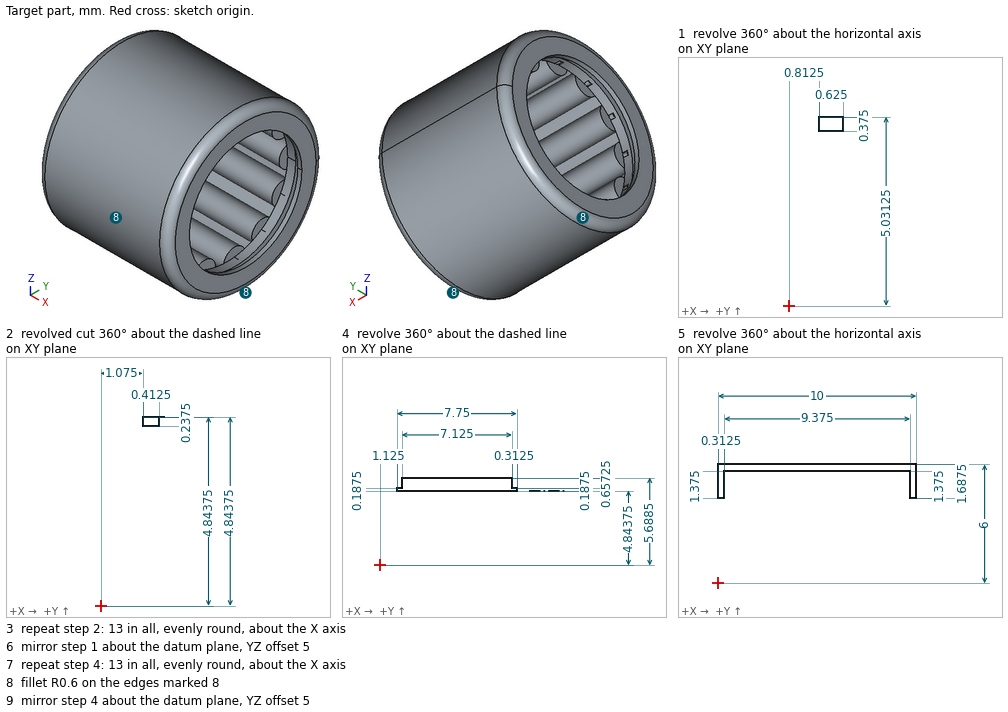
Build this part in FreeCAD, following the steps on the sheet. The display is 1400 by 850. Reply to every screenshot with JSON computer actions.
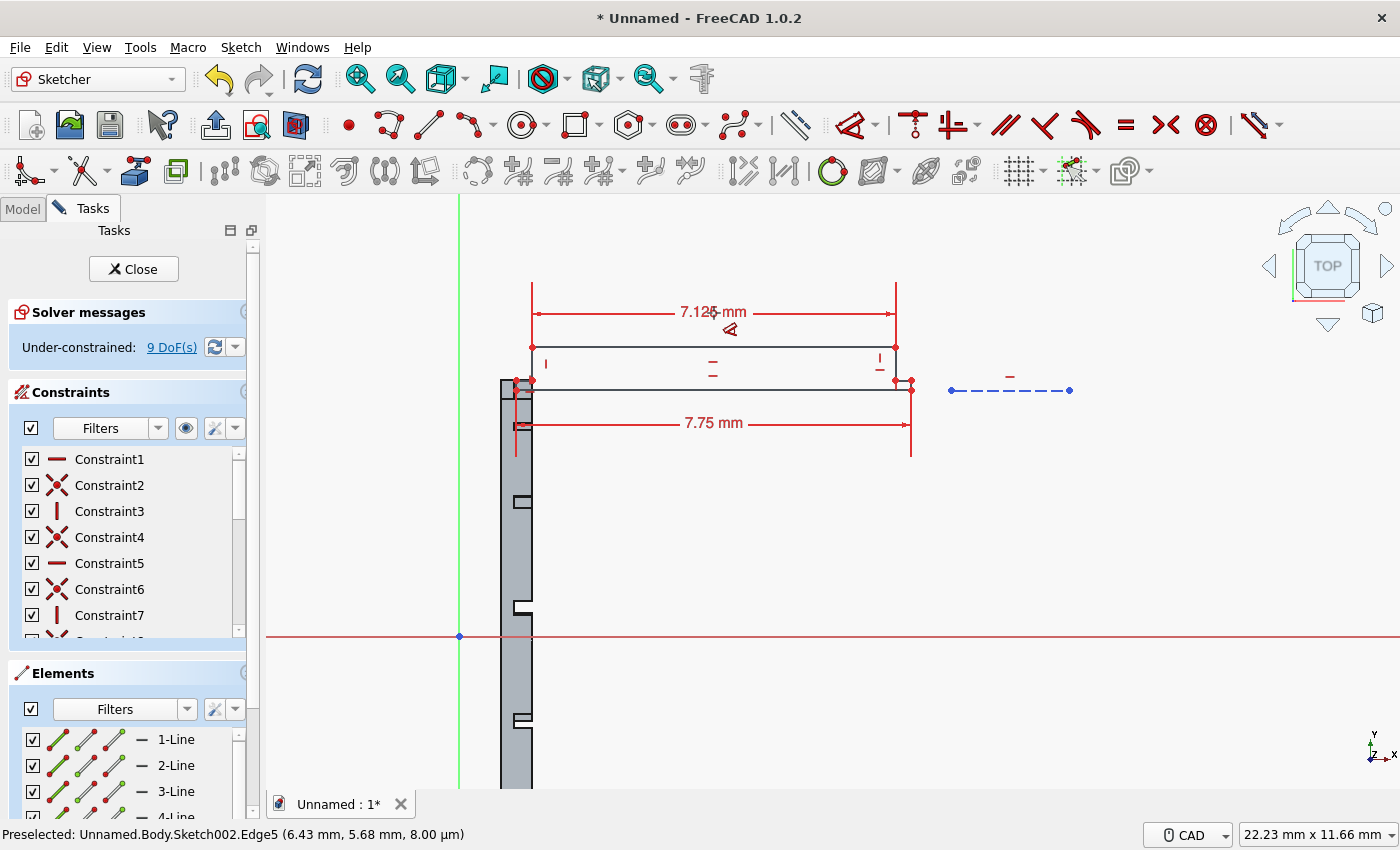
{"action": "scroll", "coordinate": [911, 386], "scroll_direction": "up", "scroll_amount": 8}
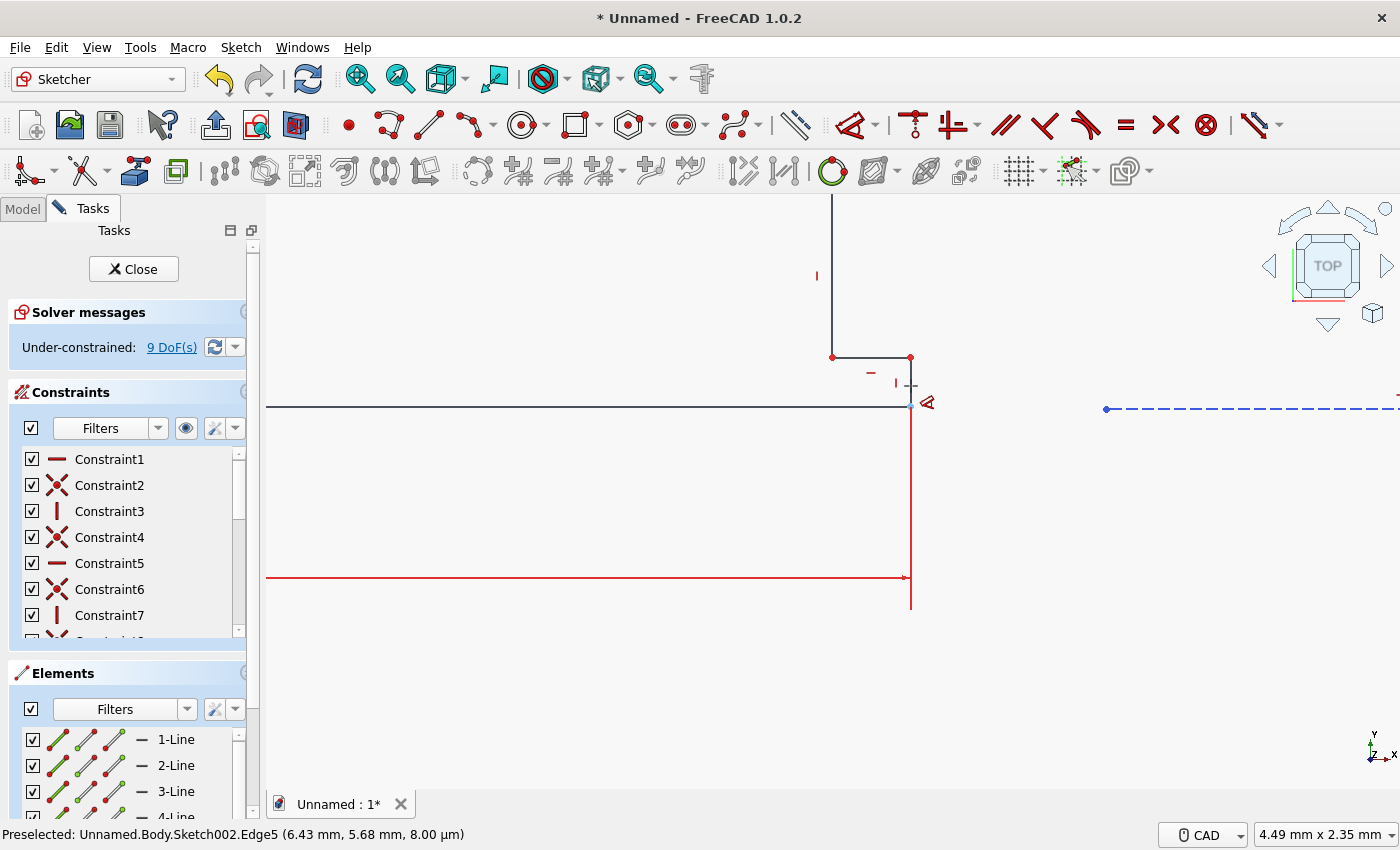
{"action": "left_click", "coordinate": [911, 382]}
{"action": "left_click", "coordinate": [945, 382]}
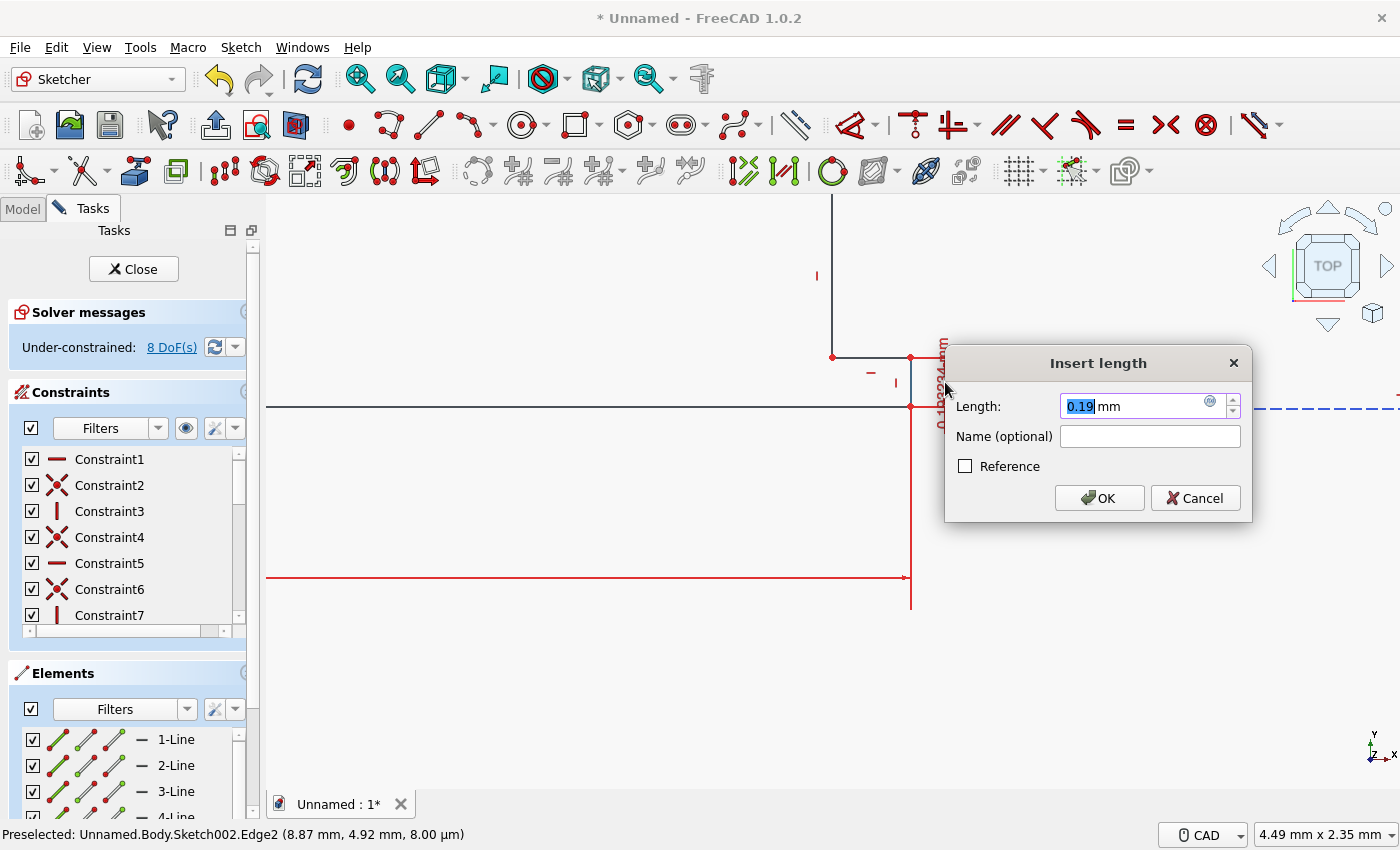
{"action": "type", "text": "0.1875"}
{"action": "key", "text": "Return"}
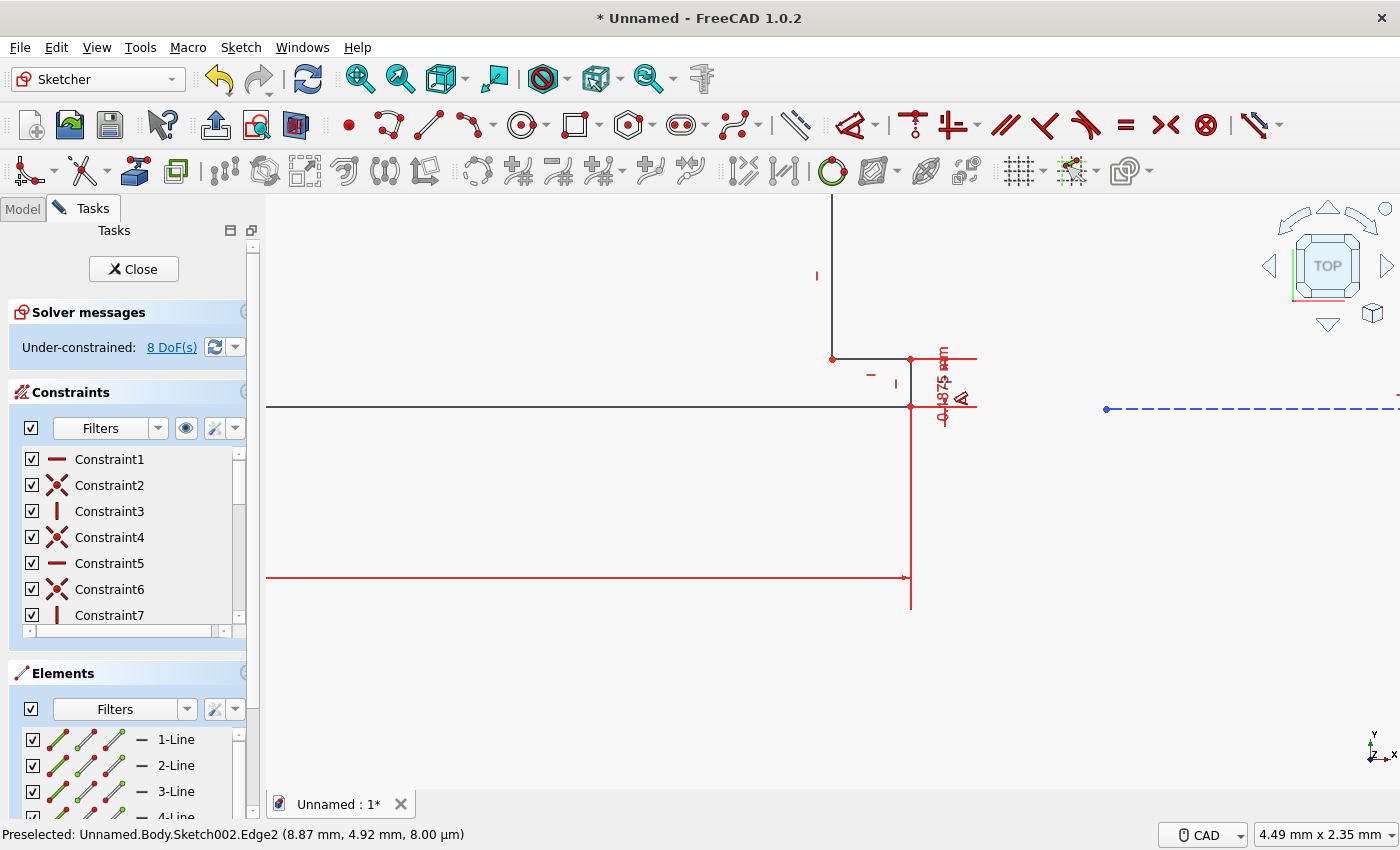
{"action": "left_click", "coordinate": [887, 359]}
{"action": "left_click", "coordinate": [872, 325]}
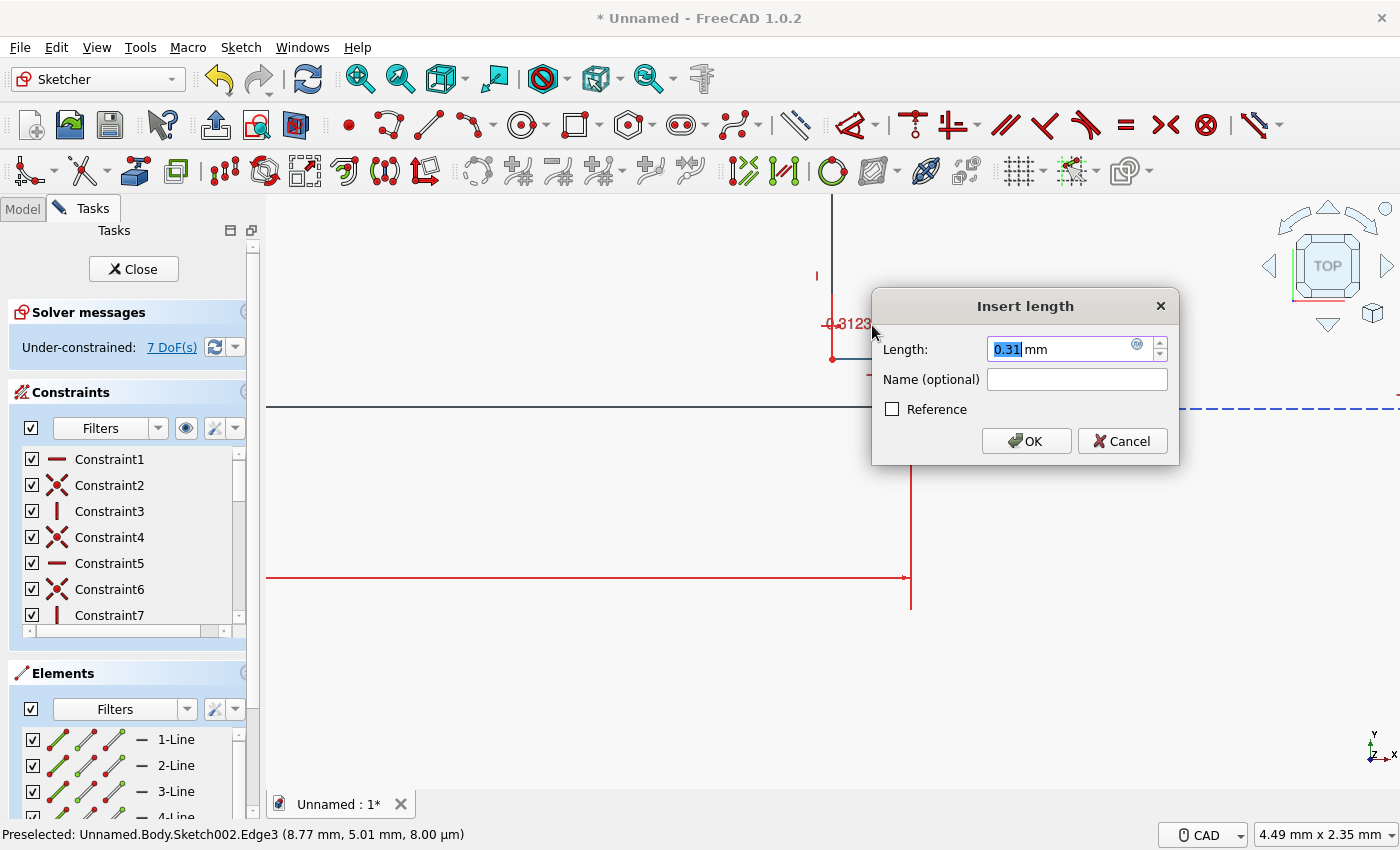
{"action": "type", "text": "0.3125"}
{"action": "key", "text": "Return"}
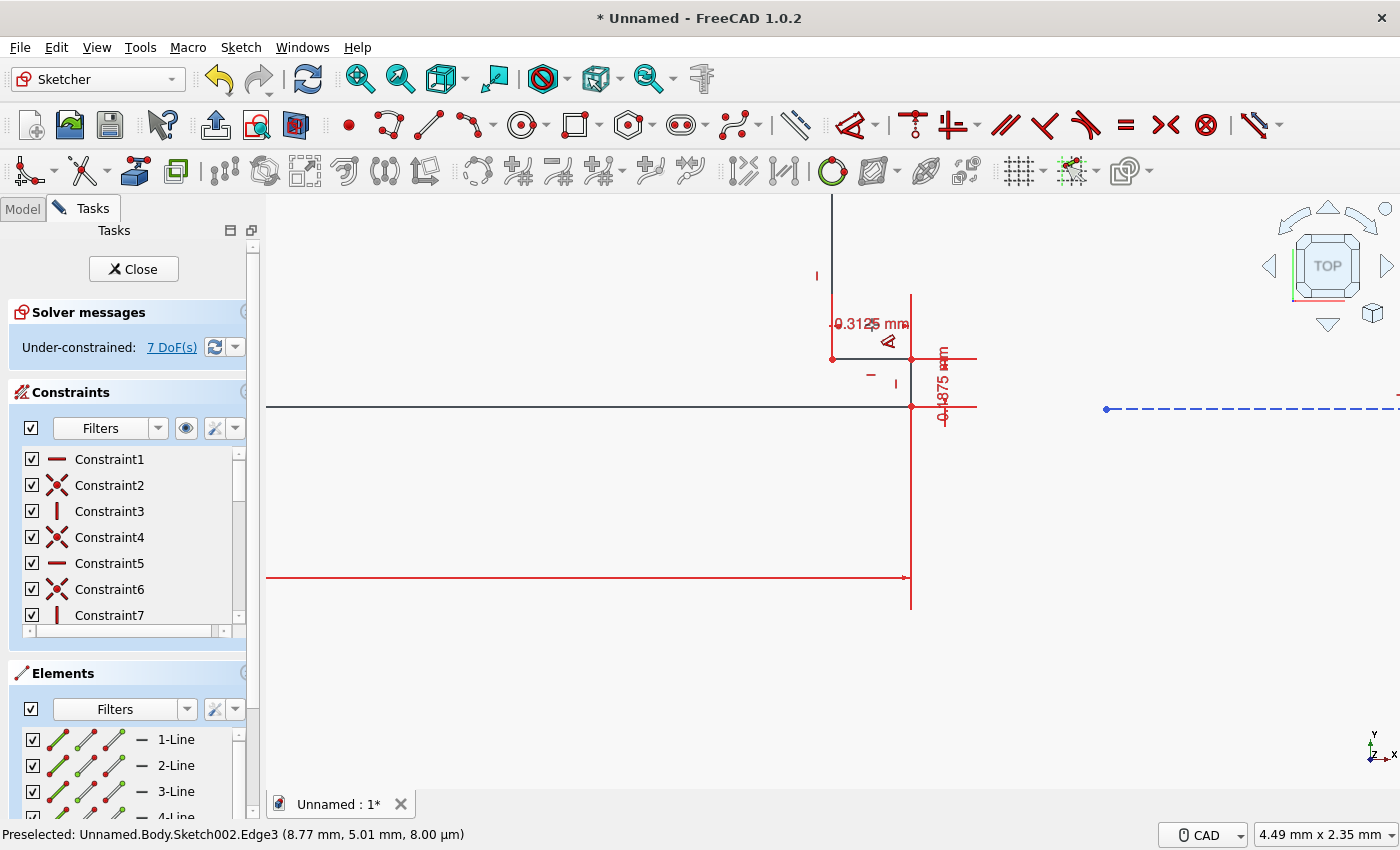
{"action": "scroll", "coordinate": [912, 386], "scroll_direction": "down", "scroll_amount": 8}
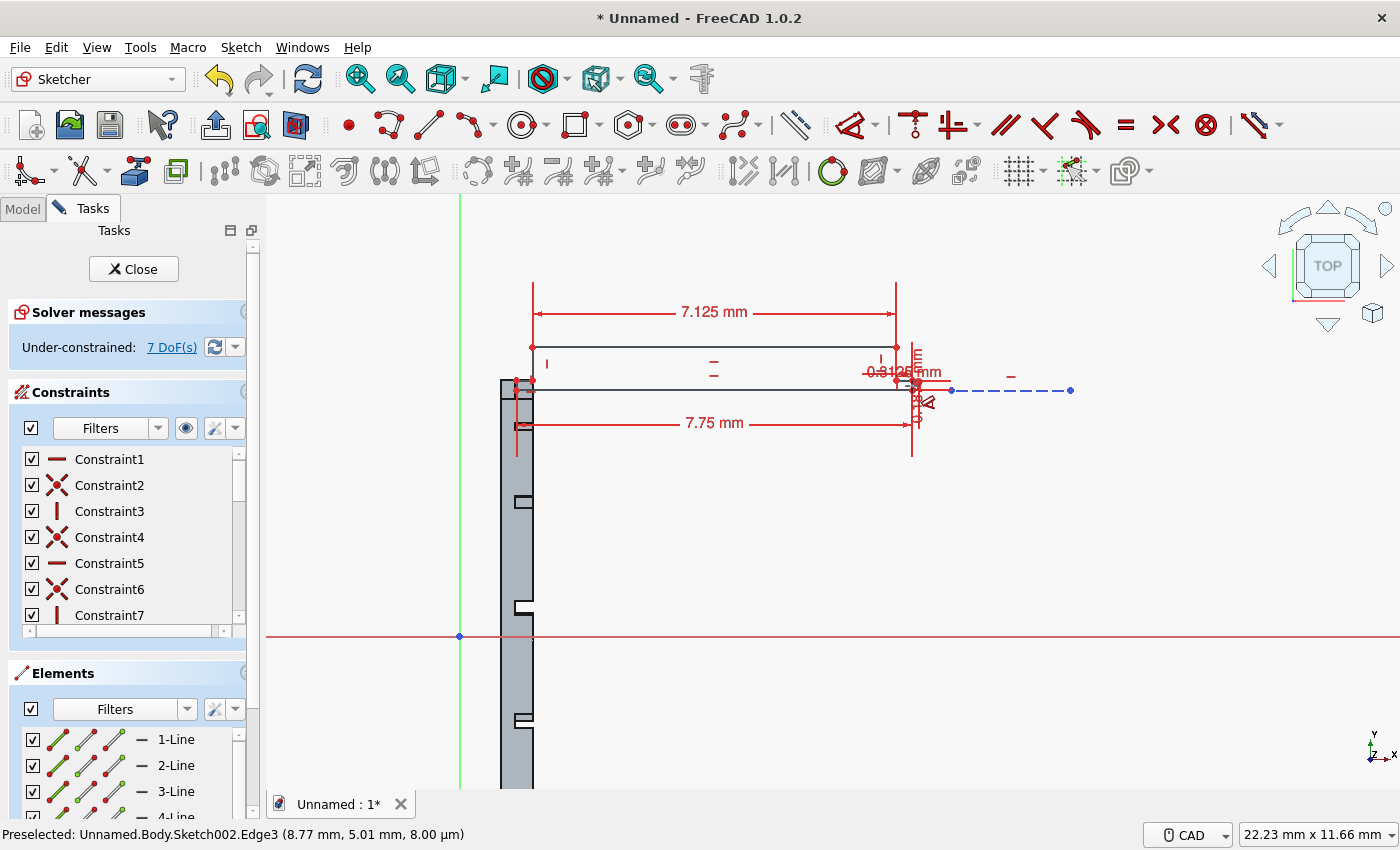
{"action": "scroll", "coordinate": [517, 384], "scroll_direction": "up", "scroll_amount": 8}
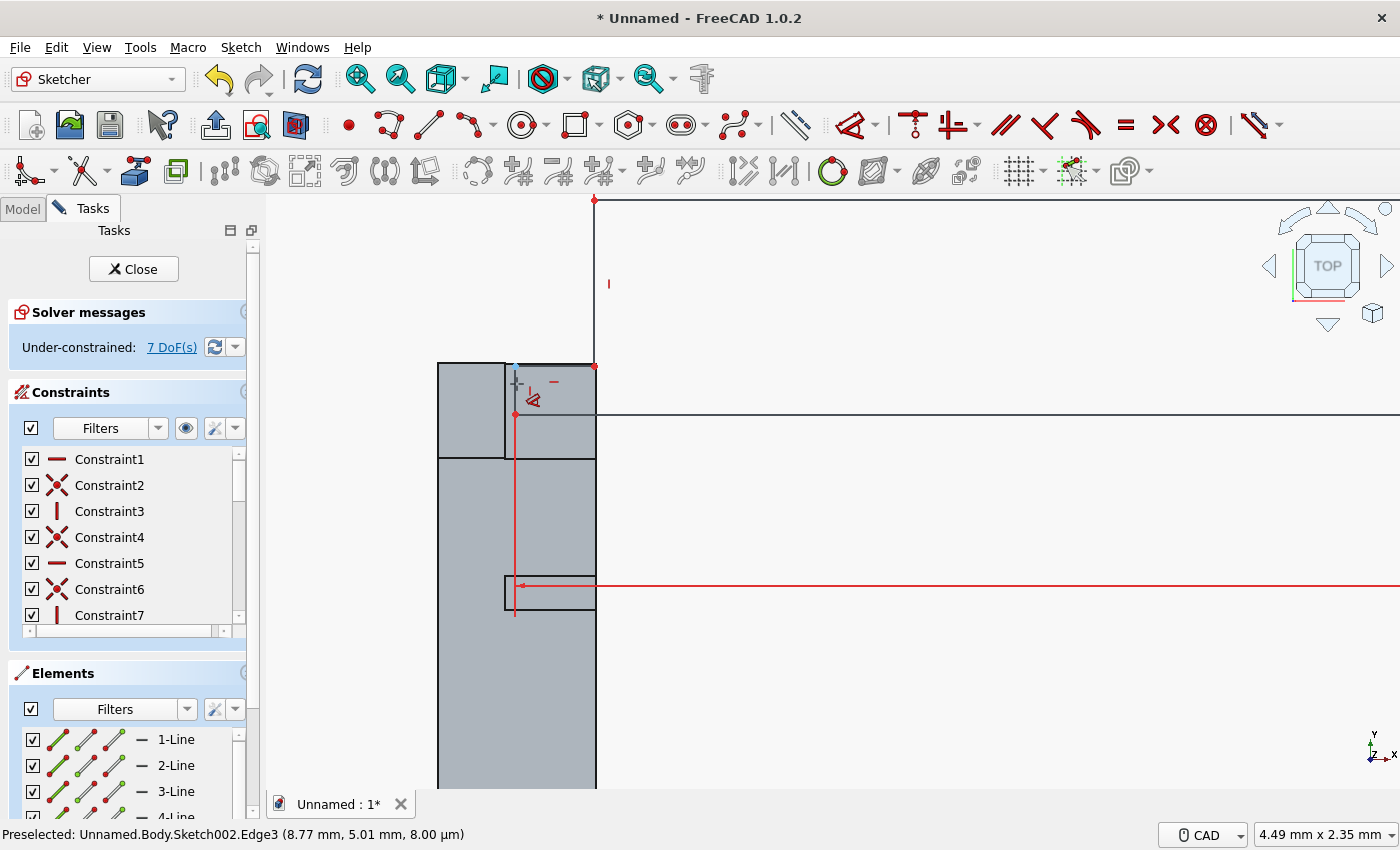
{"action": "left_click", "coordinate": [515, 381]}
{"action": "left_click", "coordinate": [481, 391]}